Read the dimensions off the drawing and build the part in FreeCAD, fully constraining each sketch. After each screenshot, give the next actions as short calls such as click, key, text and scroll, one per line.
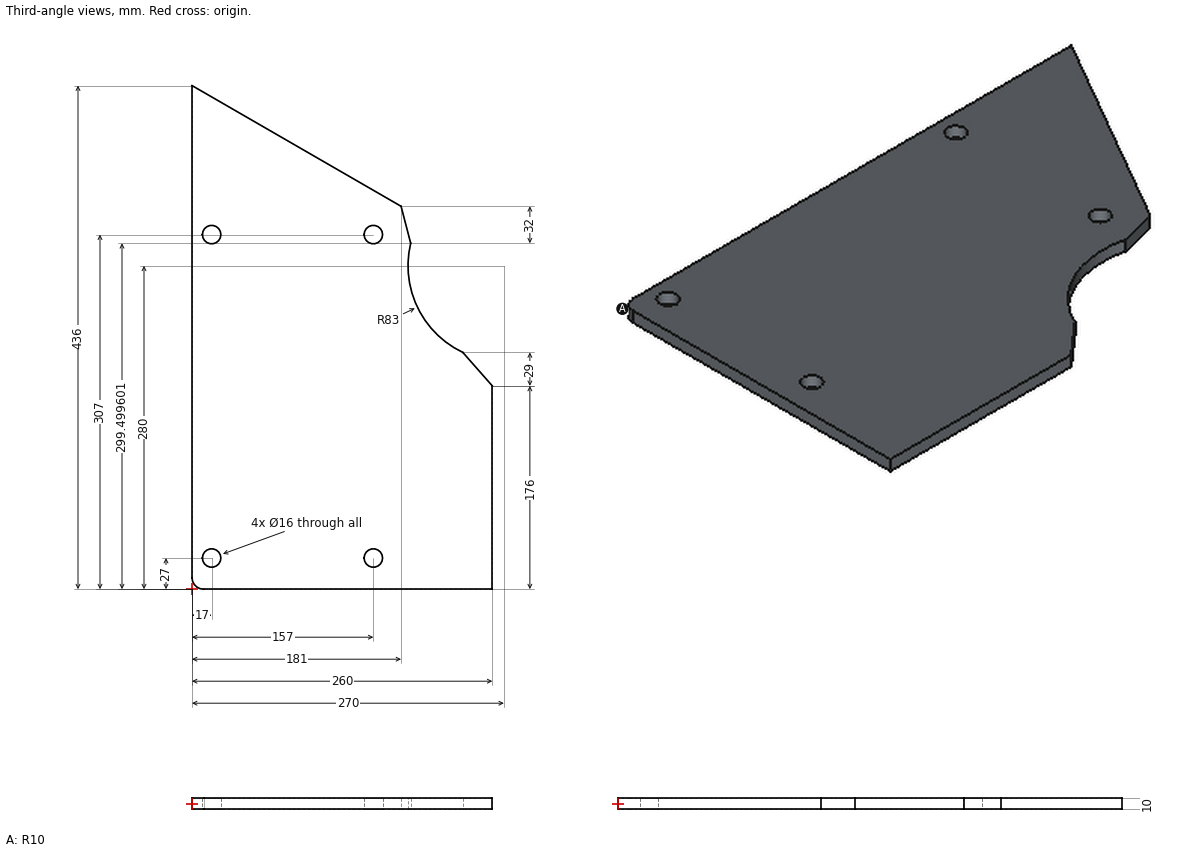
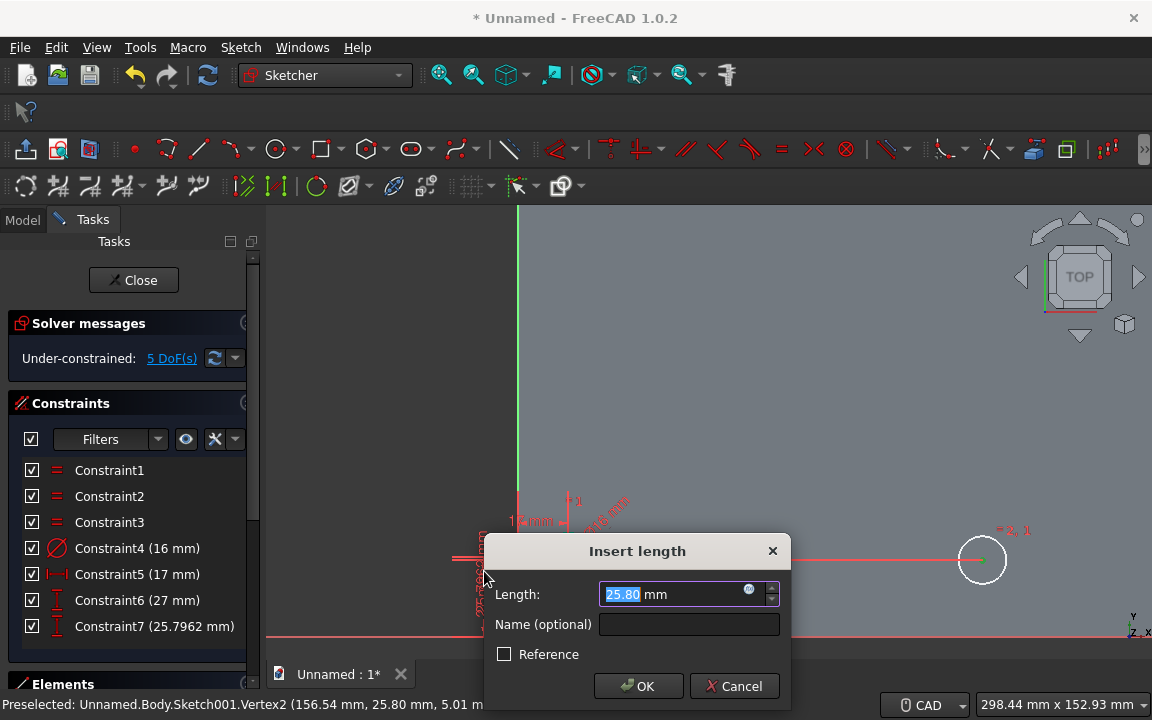
text(27)
key(Return)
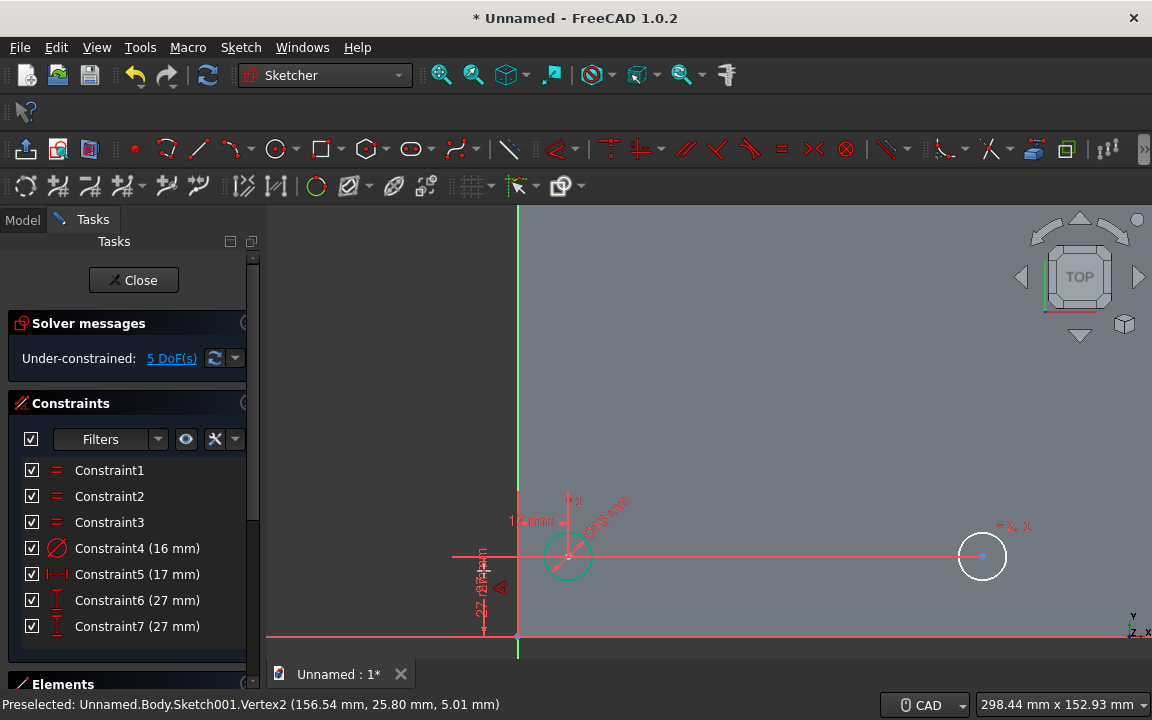
scroll(588, 545, down, 6)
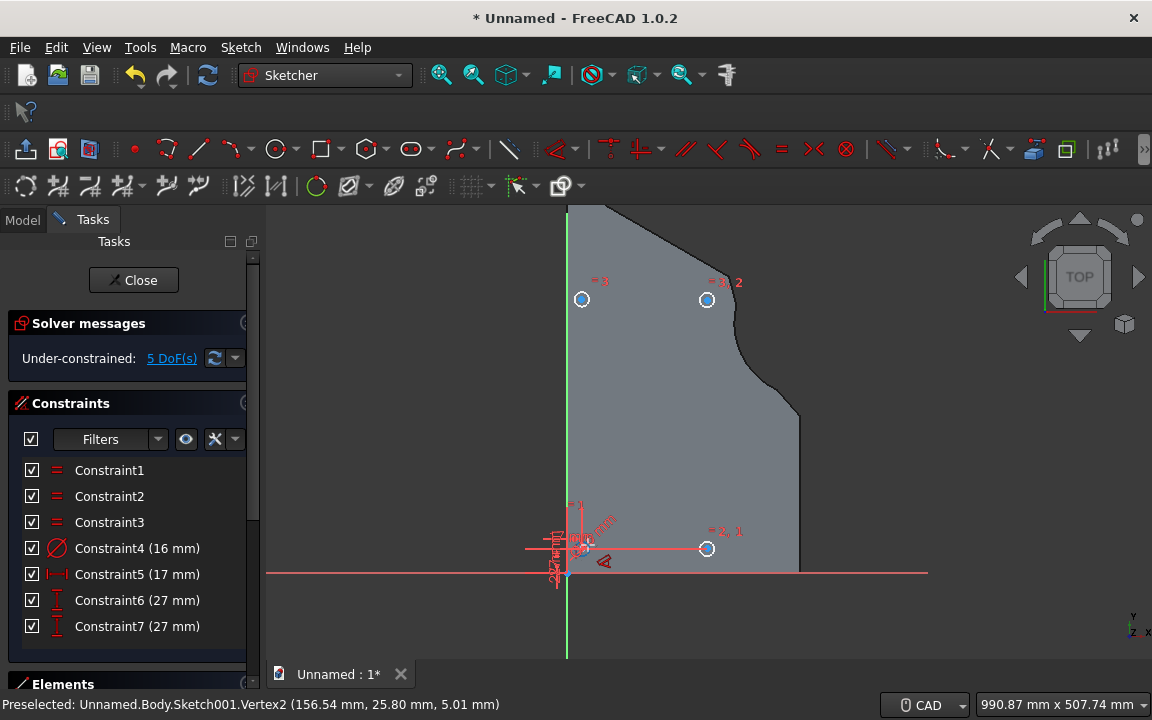
scroll(582, 299, up, 5)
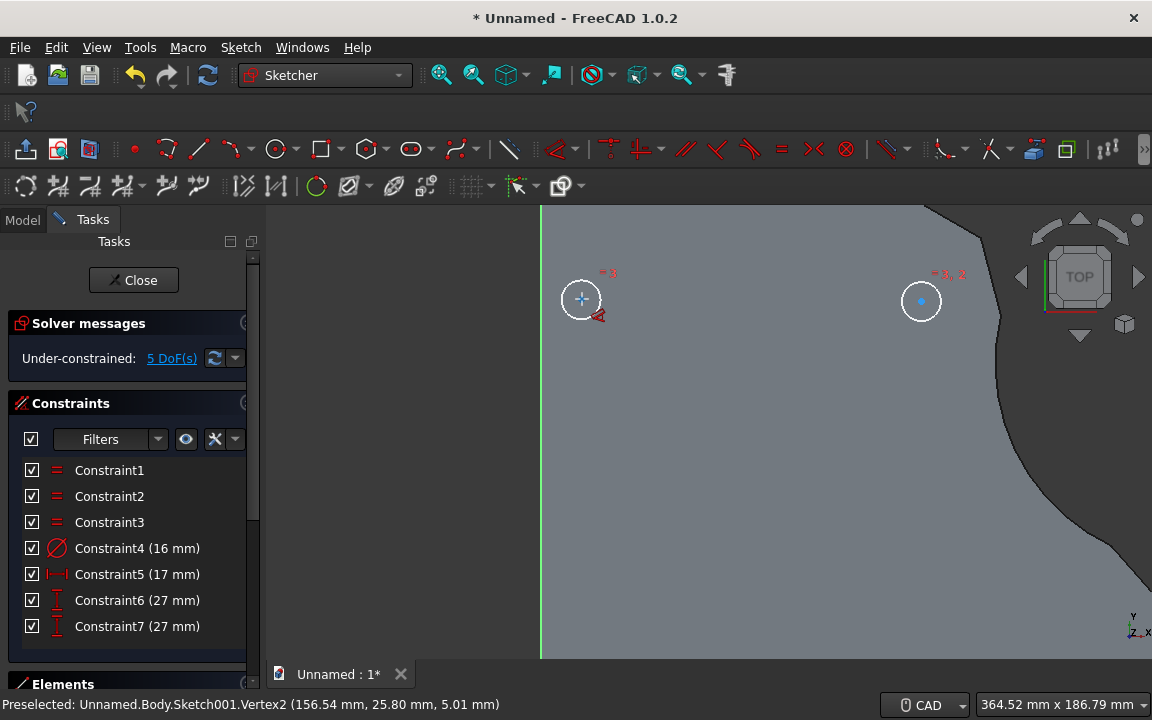
click(581, 300)
click(561, 266)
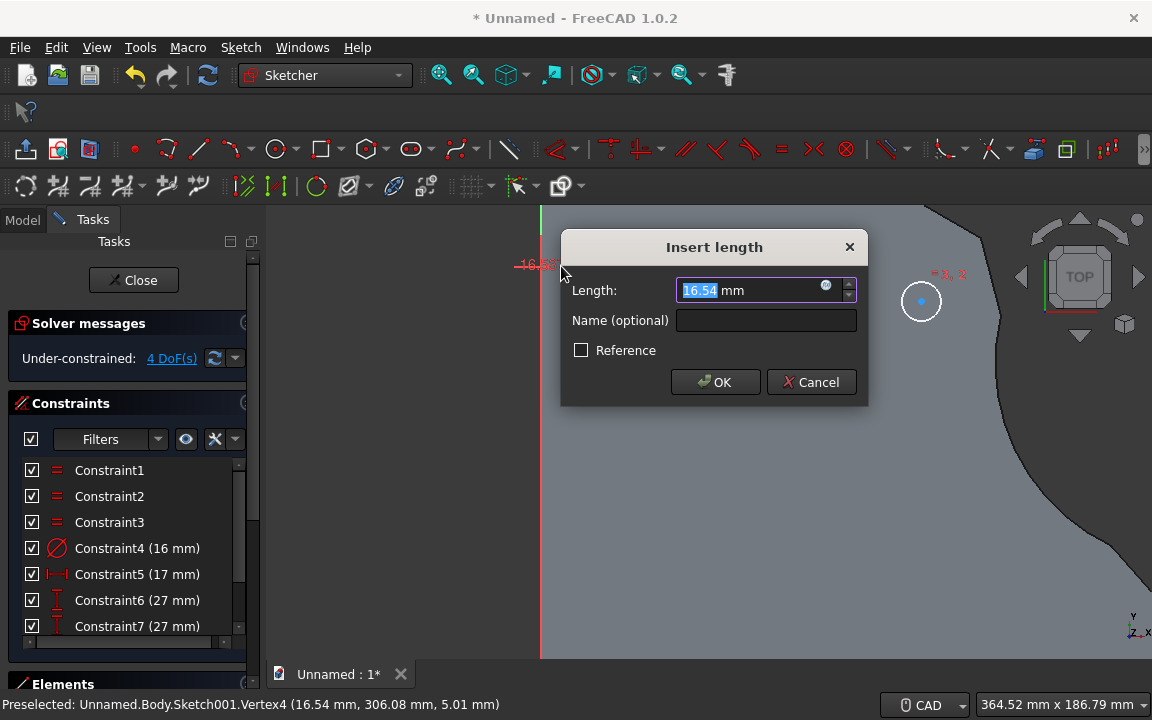
text(17)
key(Return)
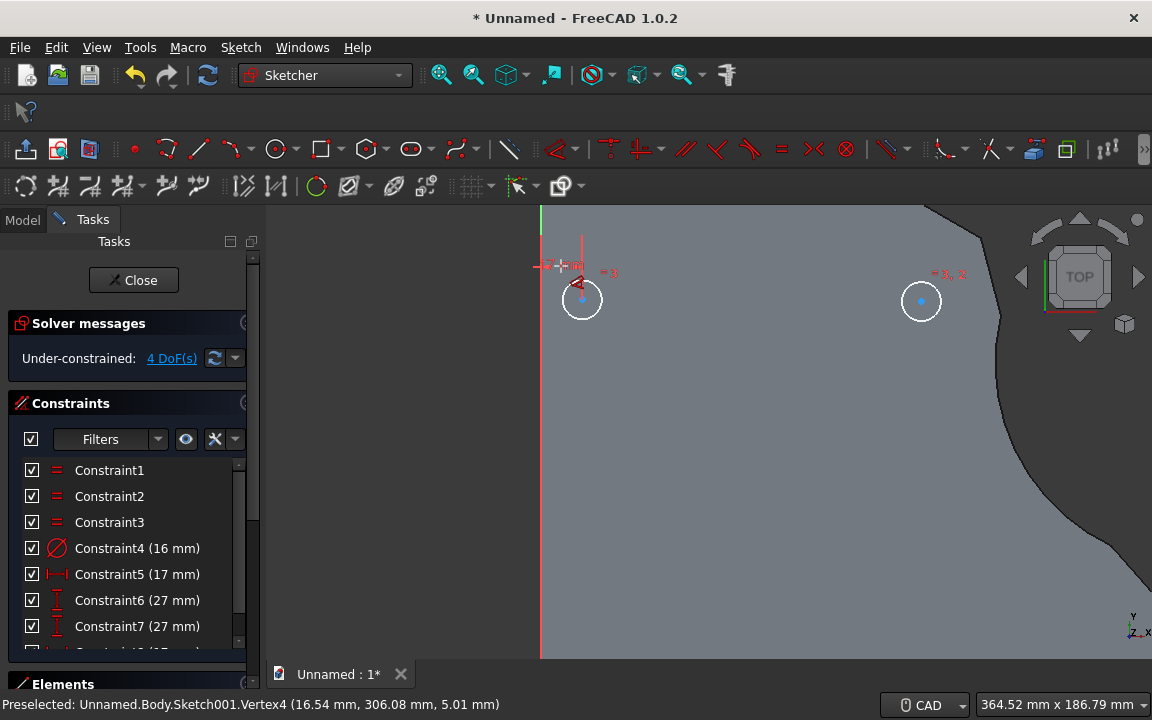
scroll(582, 299, down, 5)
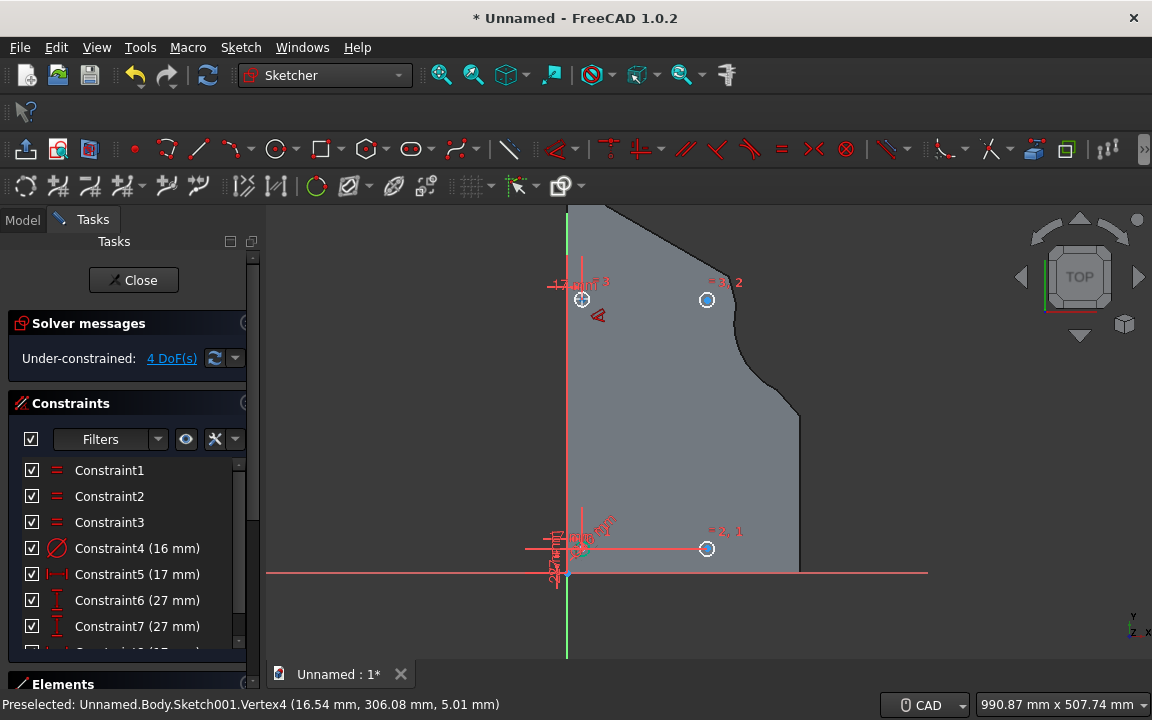
click(707, 549)
click(637, 607)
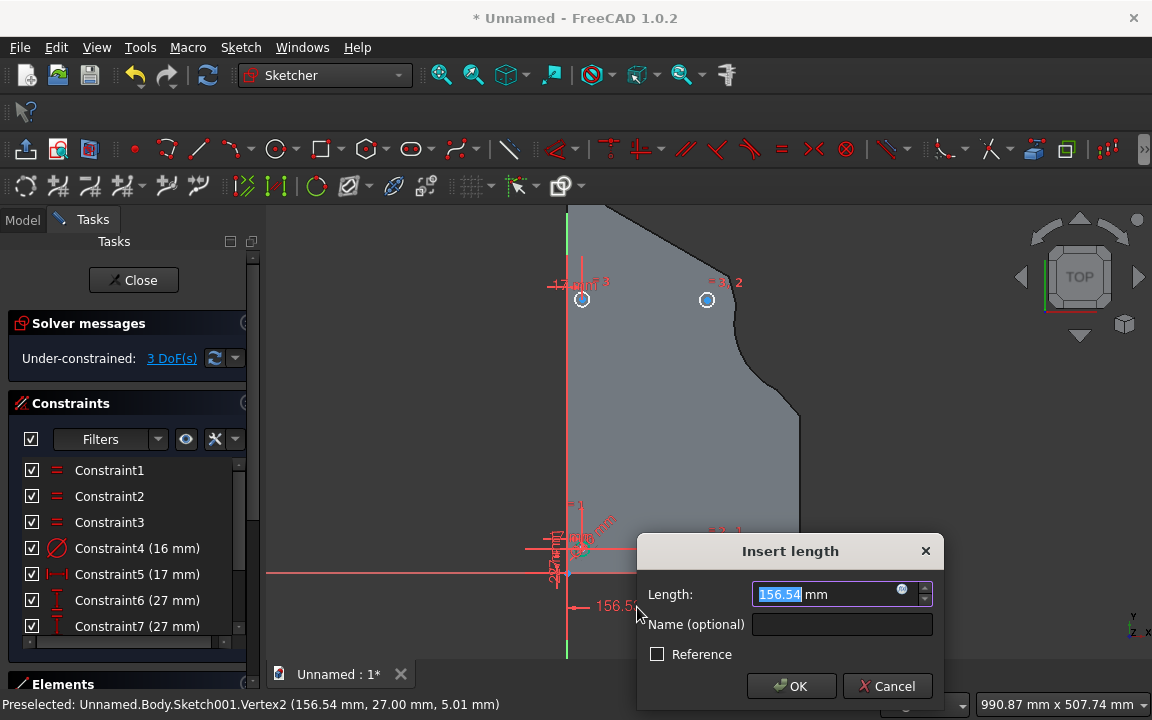
text(157)
key(Return)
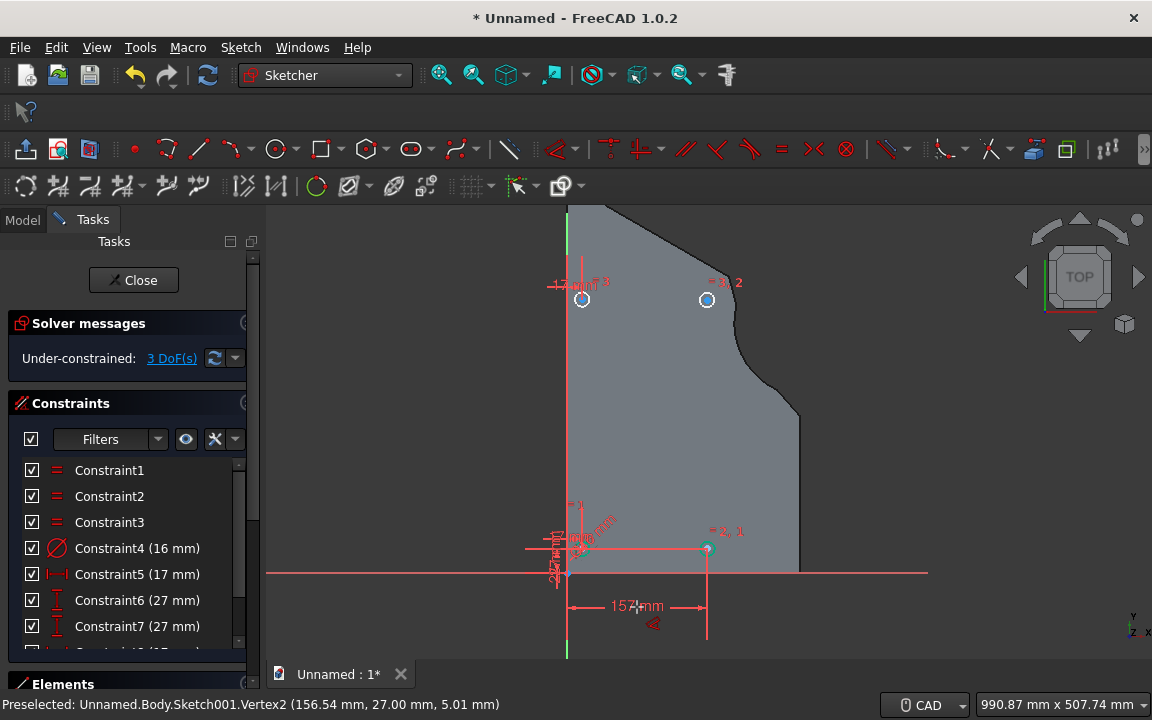
click(707, 300)
click(637, 266)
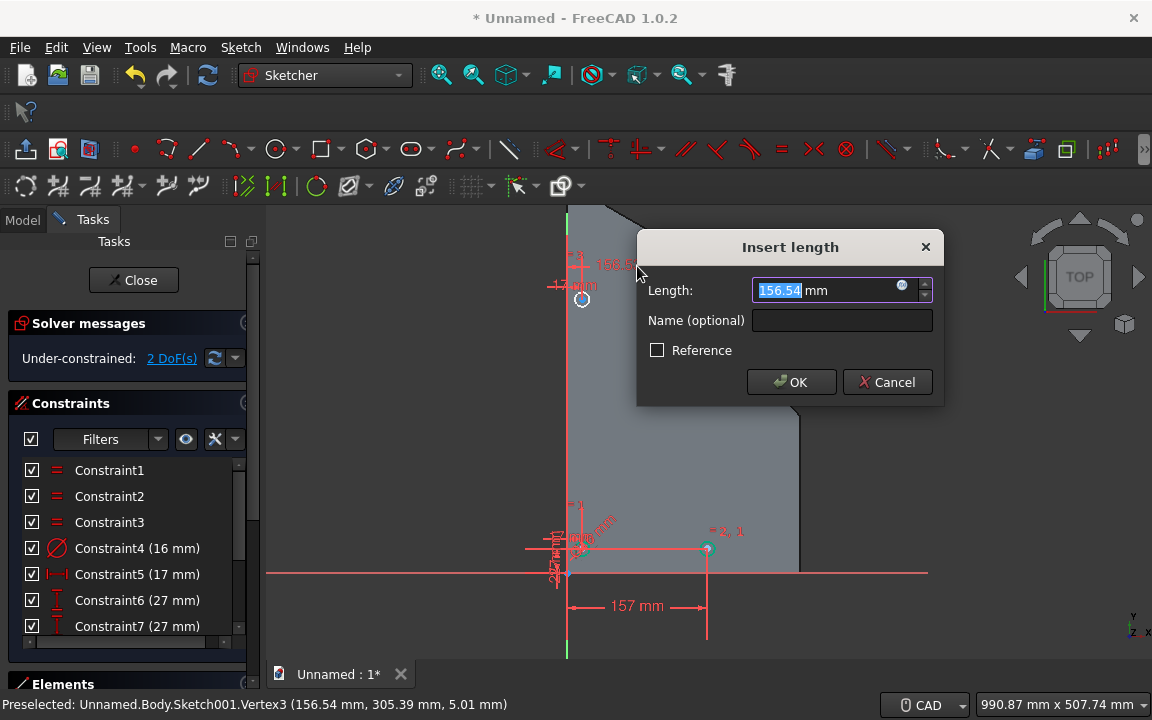
text(157)
key(Return)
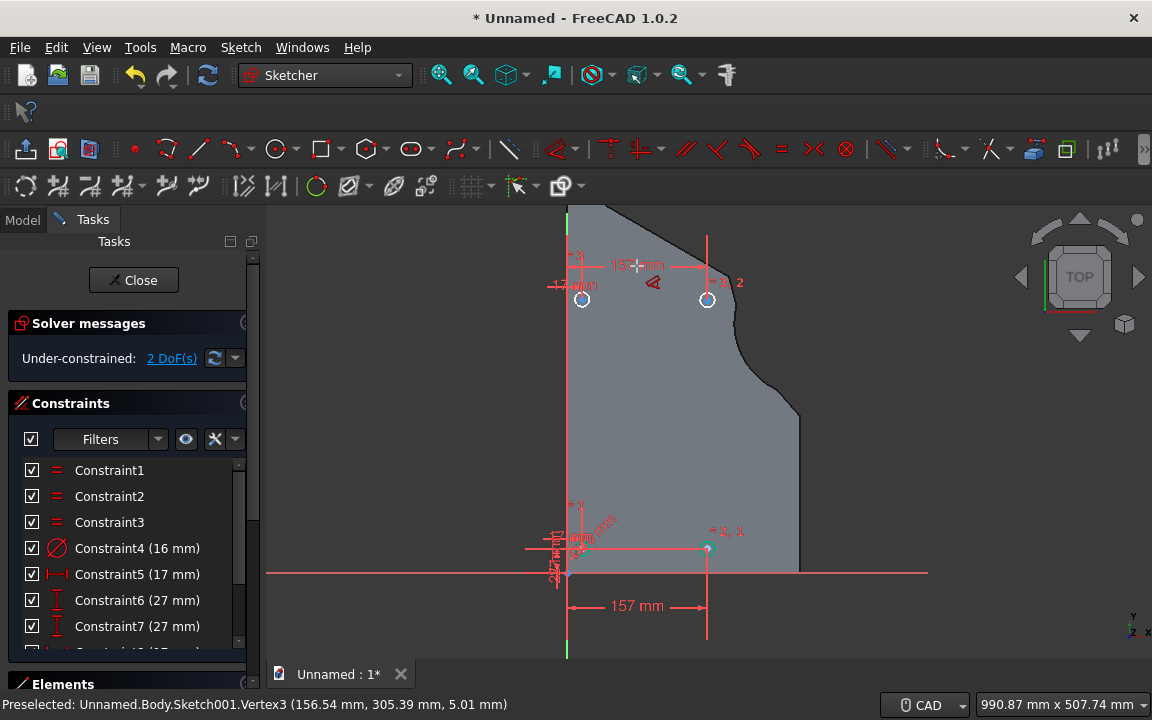
click(707, 300)
click(533, 437)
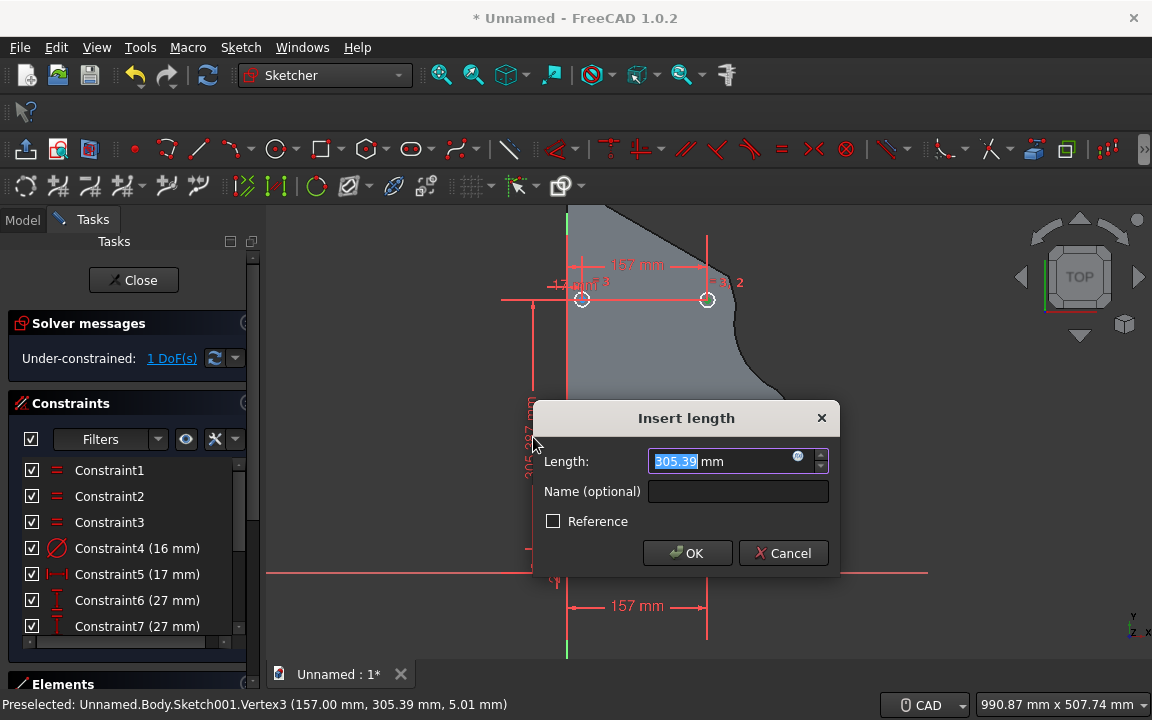
text(307)
key(Return)